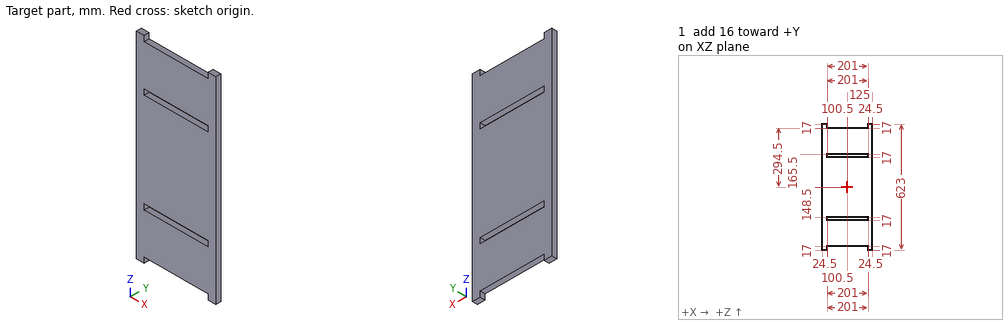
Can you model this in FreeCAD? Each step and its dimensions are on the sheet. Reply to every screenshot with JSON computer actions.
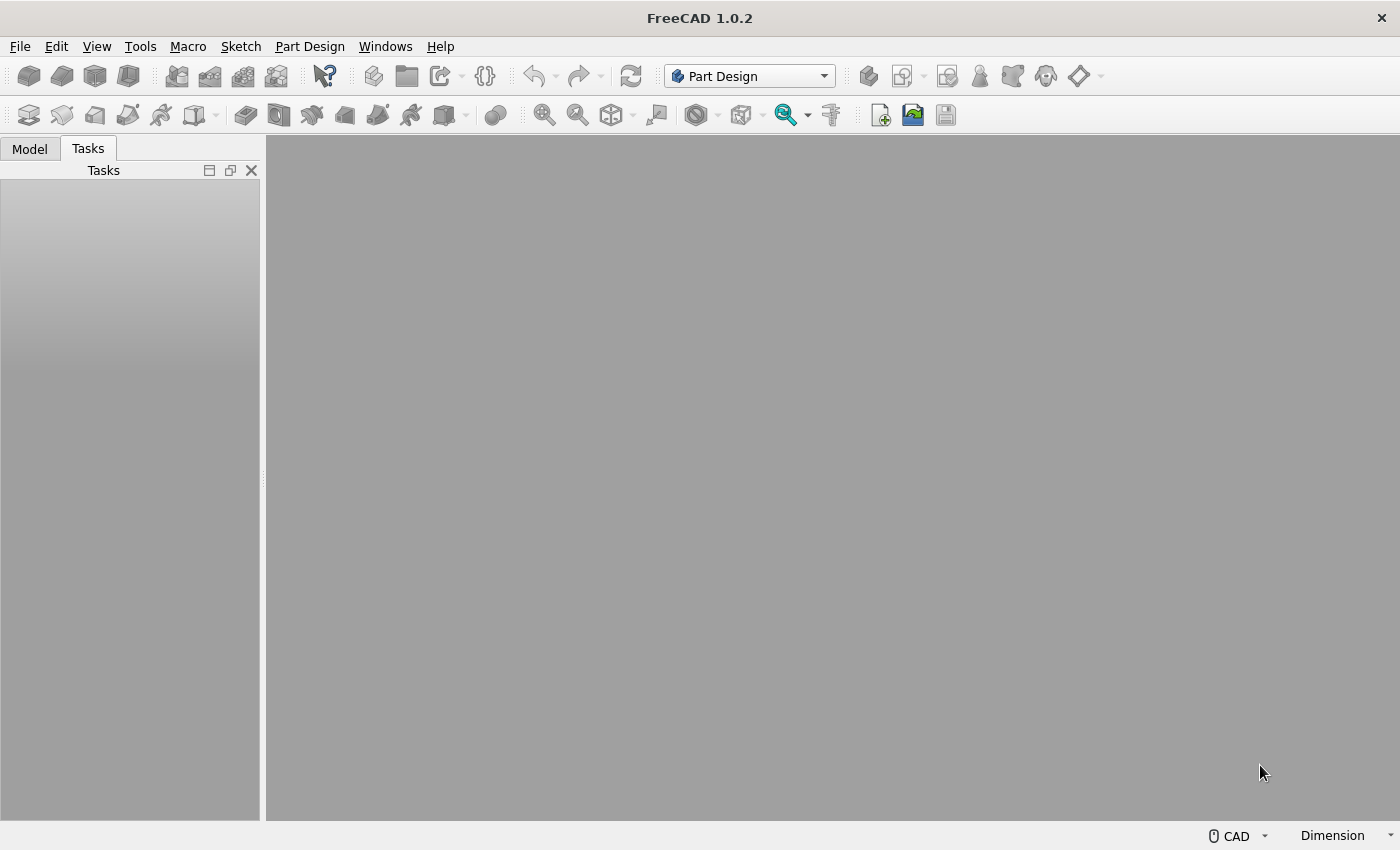
{"action": "left_click", "coordinate": [880, 116]}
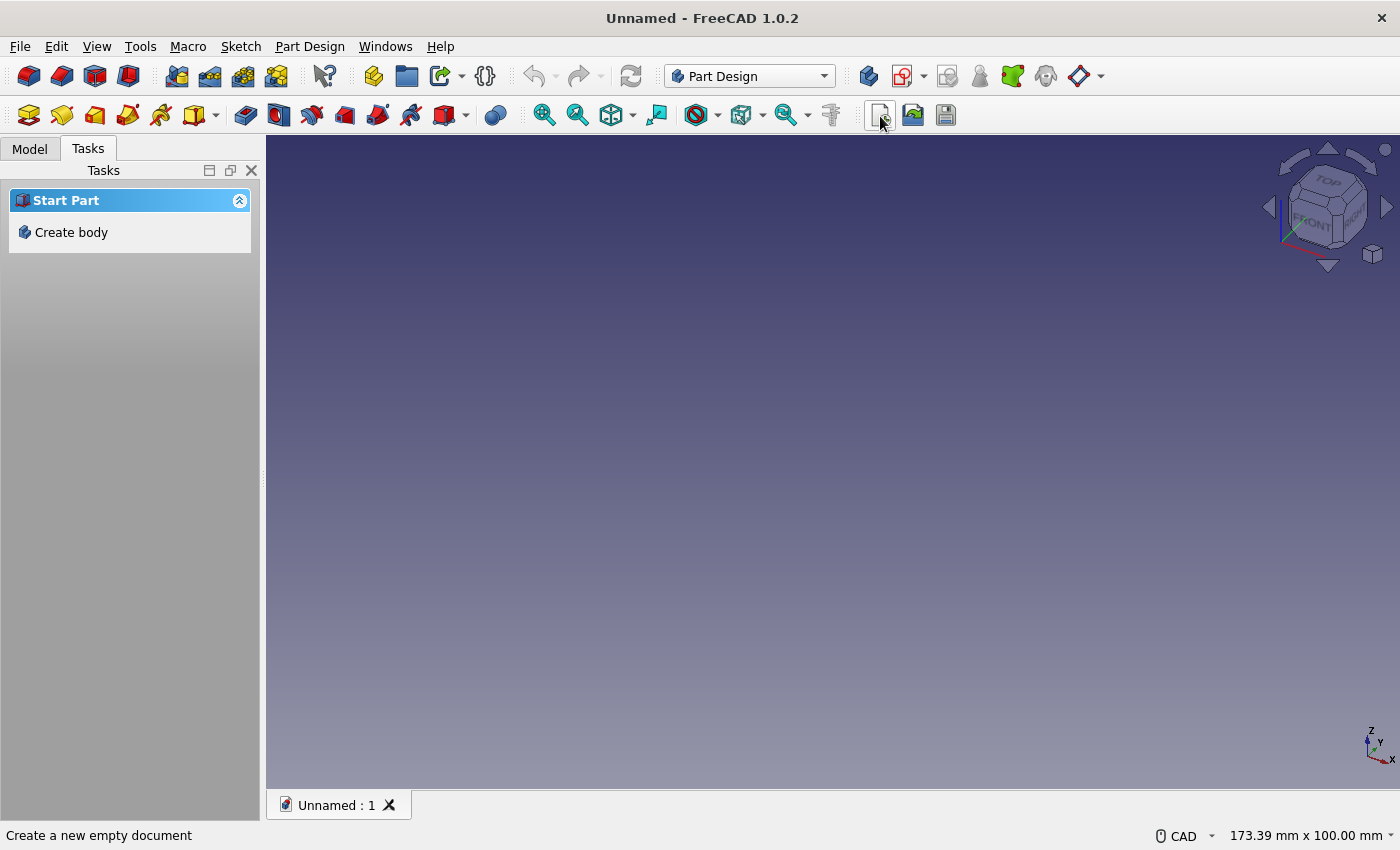
{"action": "left_click", "coordinate": [902, 76]}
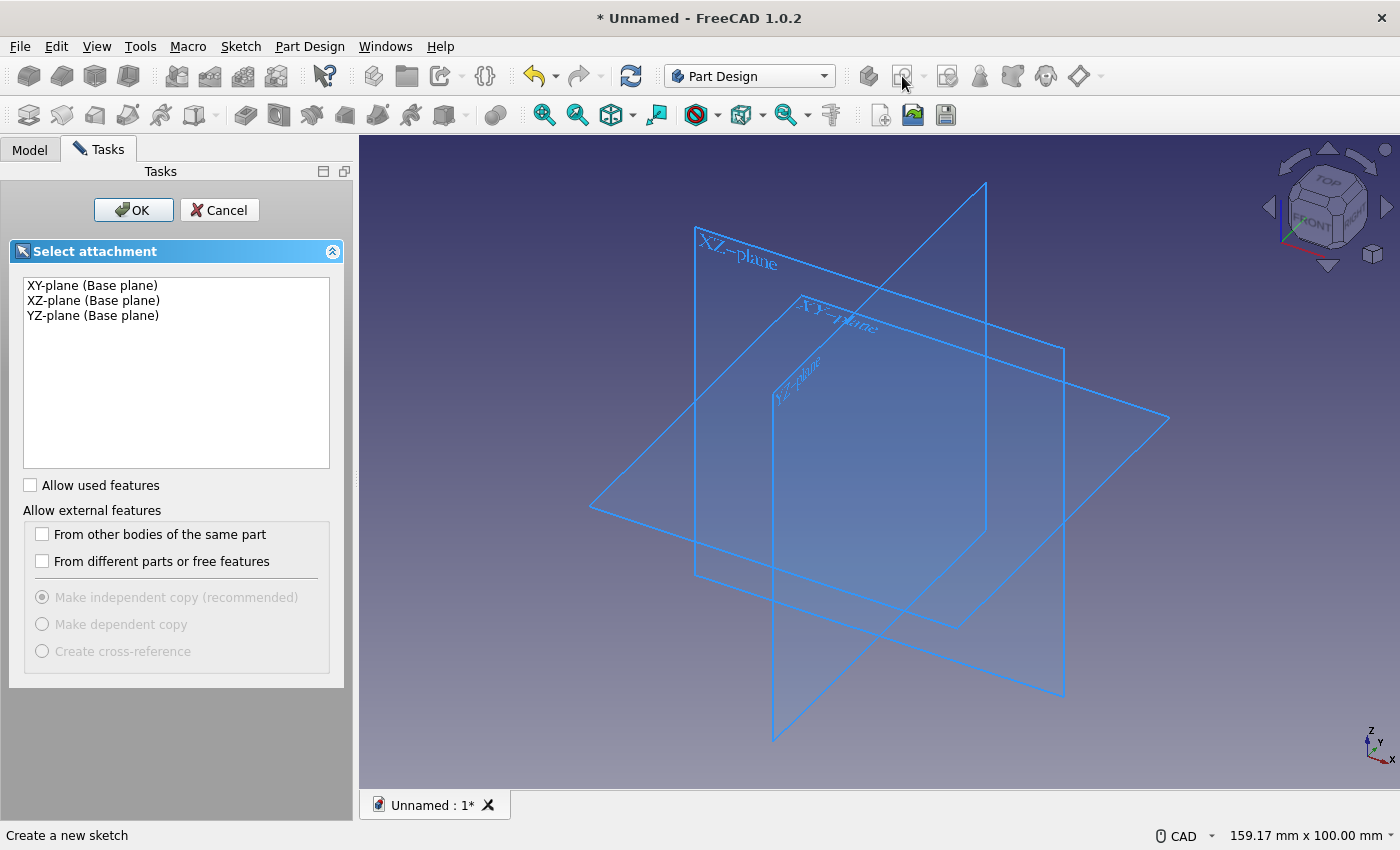
{"action": "left_click", "coordinate": [84, 300]}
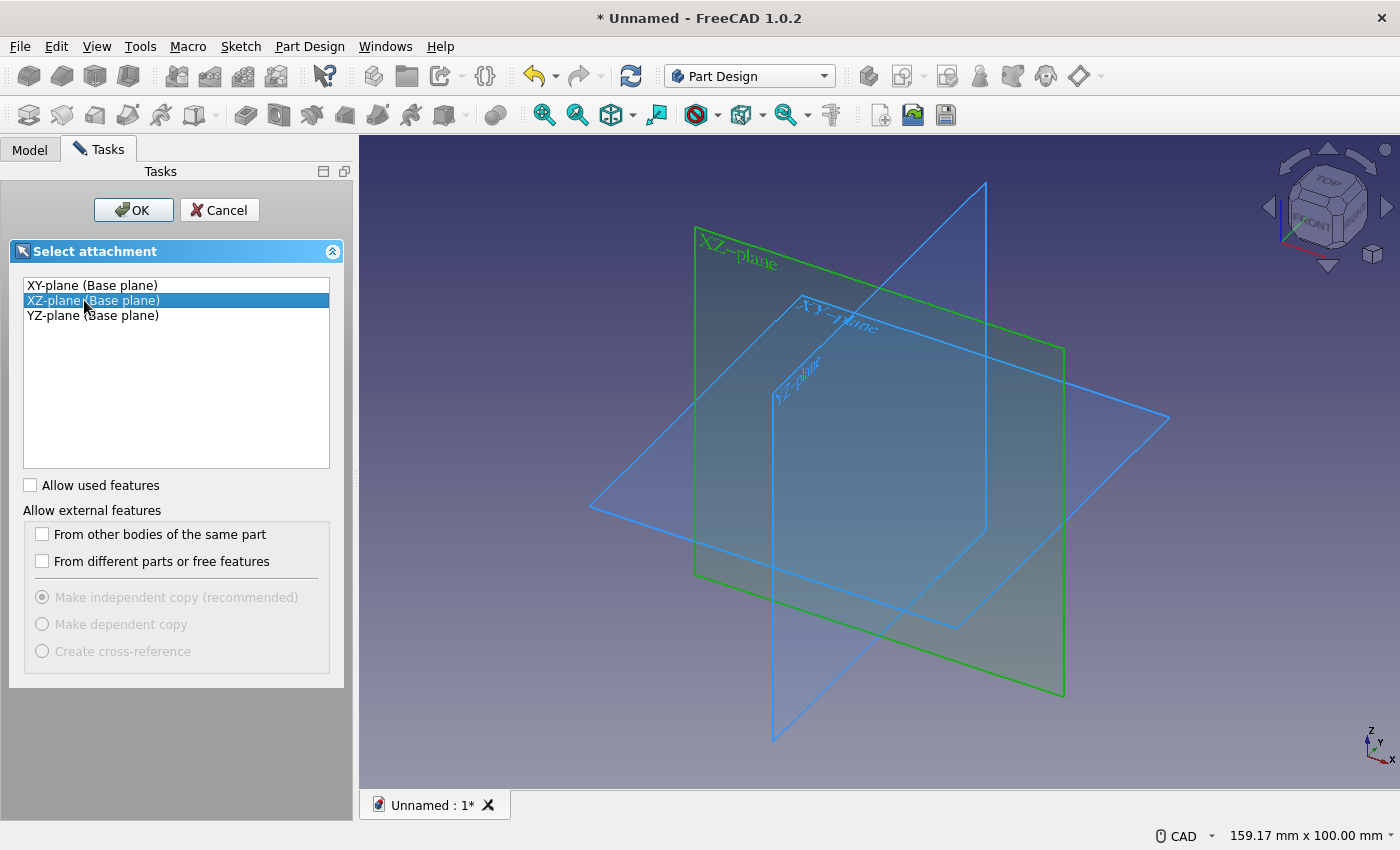
{"action": "left_click", "coordinate": [134, 210]}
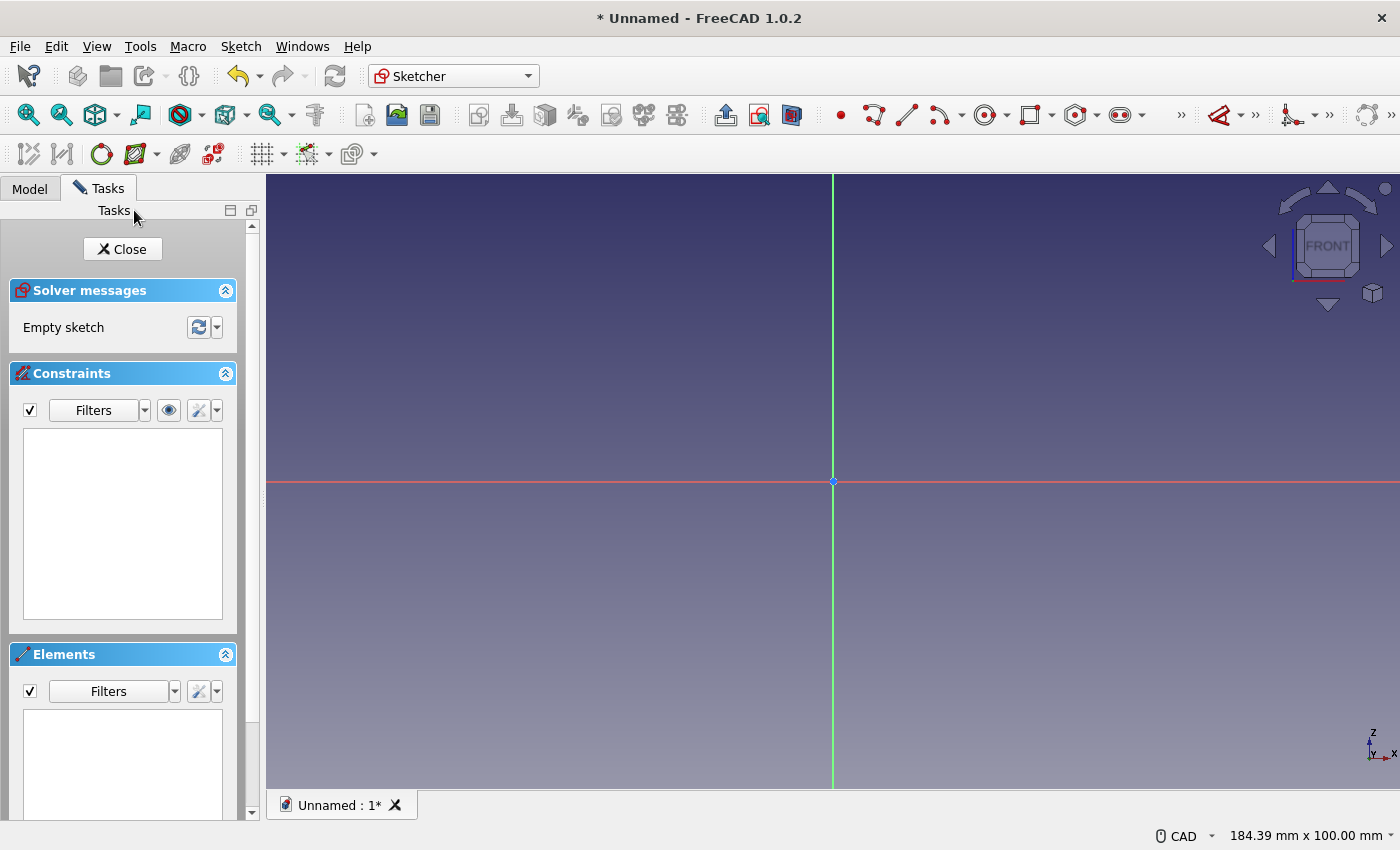
{"action": "scroll", "coordinate": [756, 482], "scroll_direction": "down", "scroll_amount": 11}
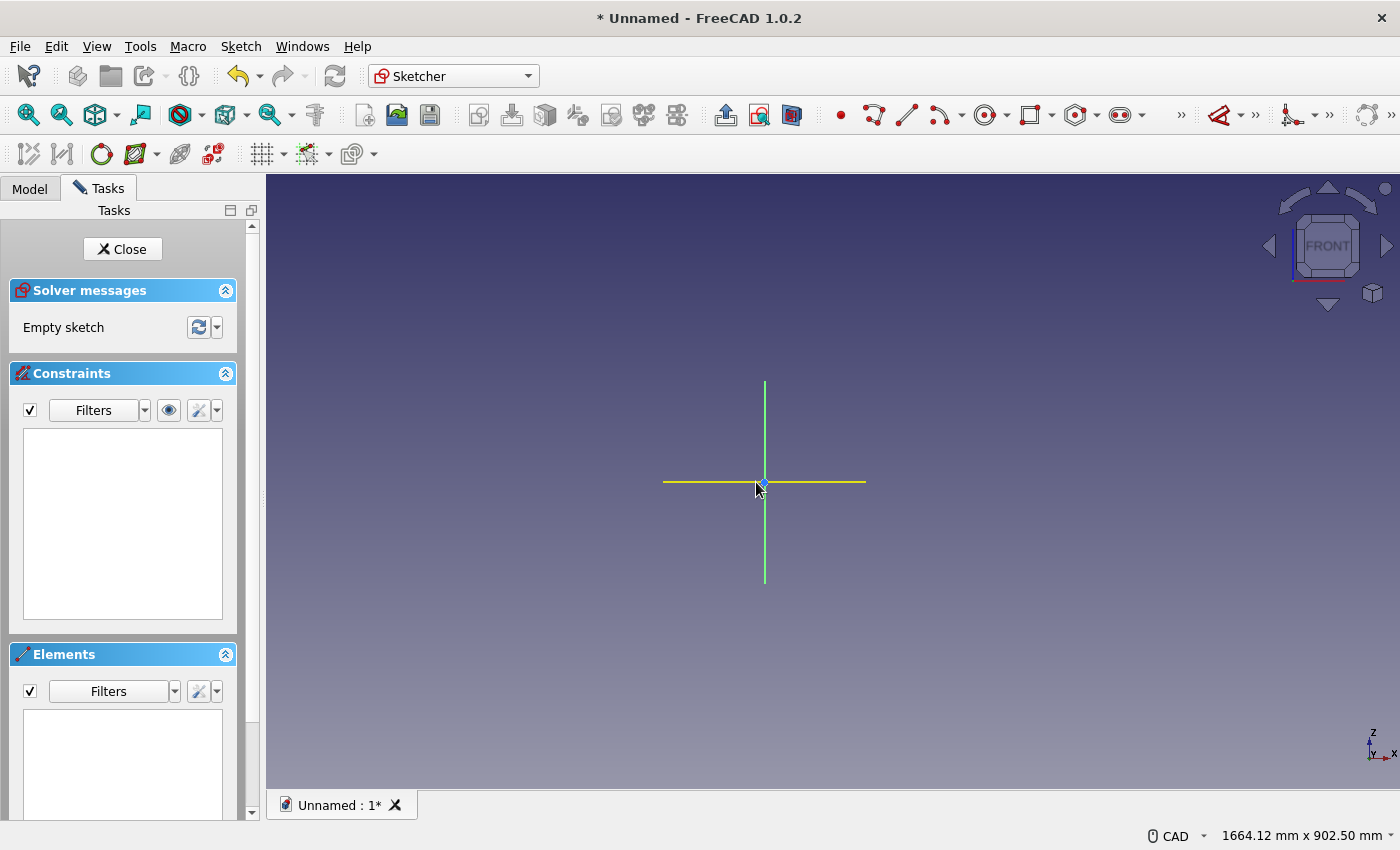
{"action": "left_click", "coordinate": [874, 116]}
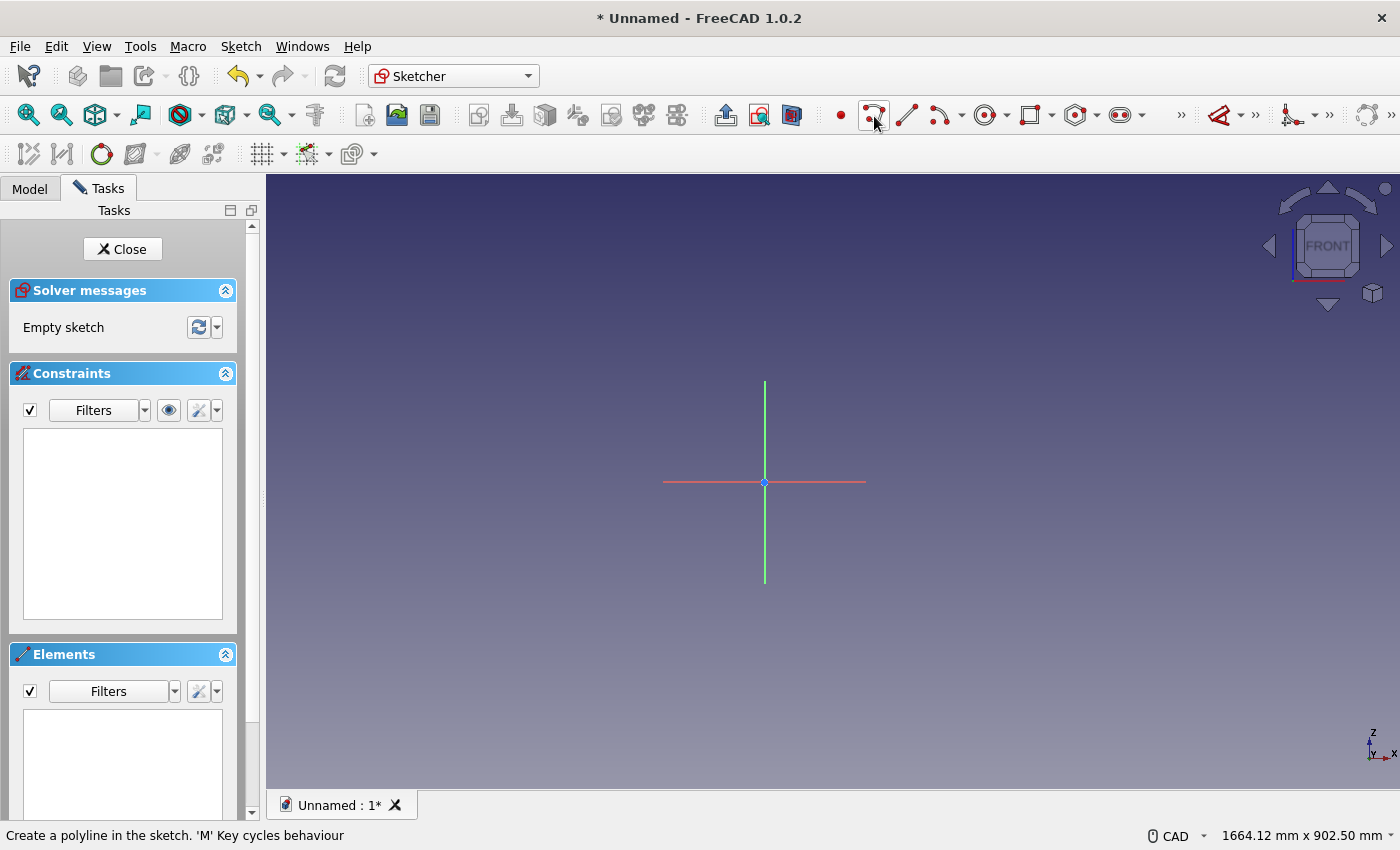
{"action": "left_click", "coordinate": [696, 282]}
{"action": "left_click", "coordinate": [833, 282]}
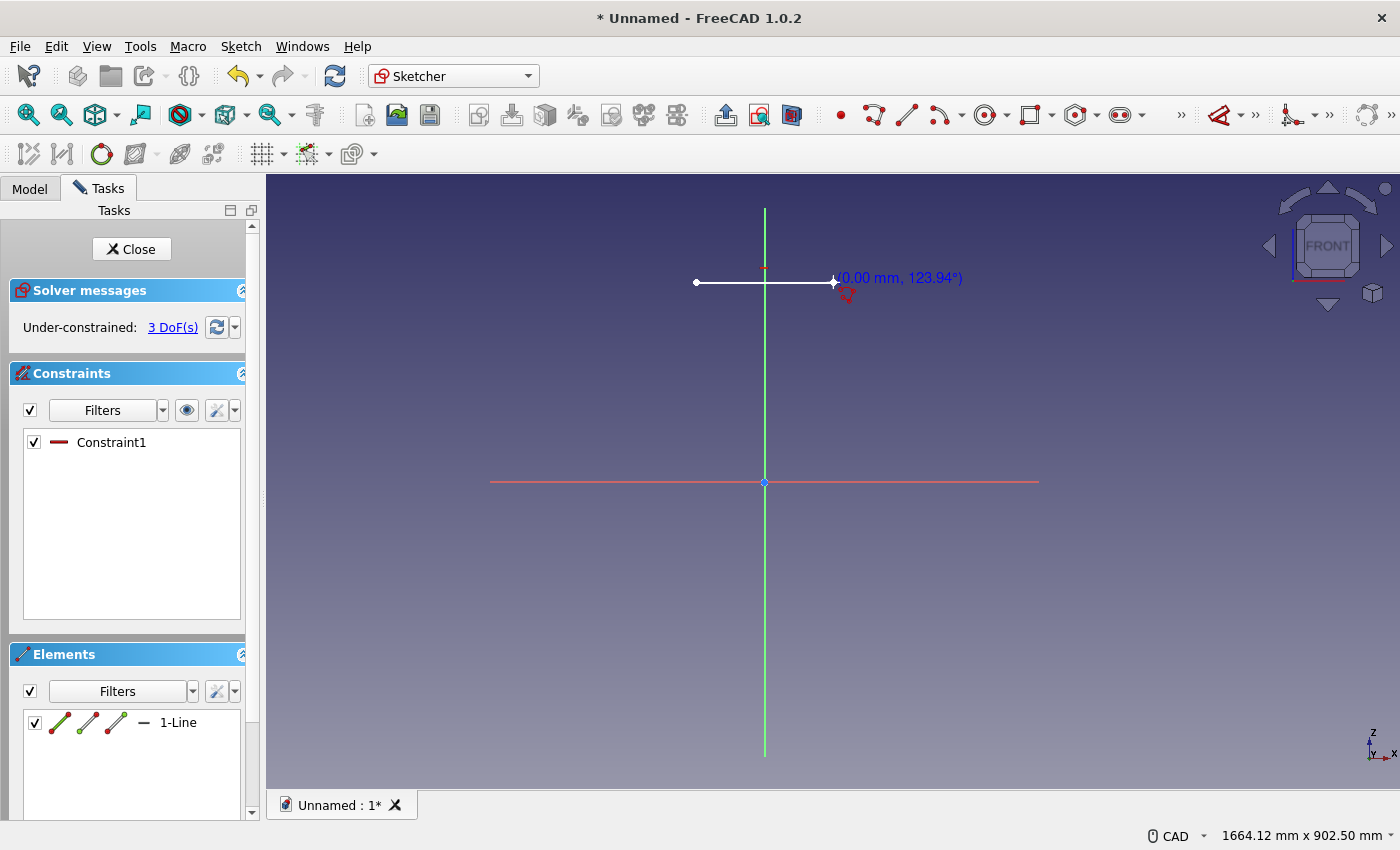
{"action": "scroll", "coordinate": [833, 270], "scroll_direction": "up", "scroll_amount": 2}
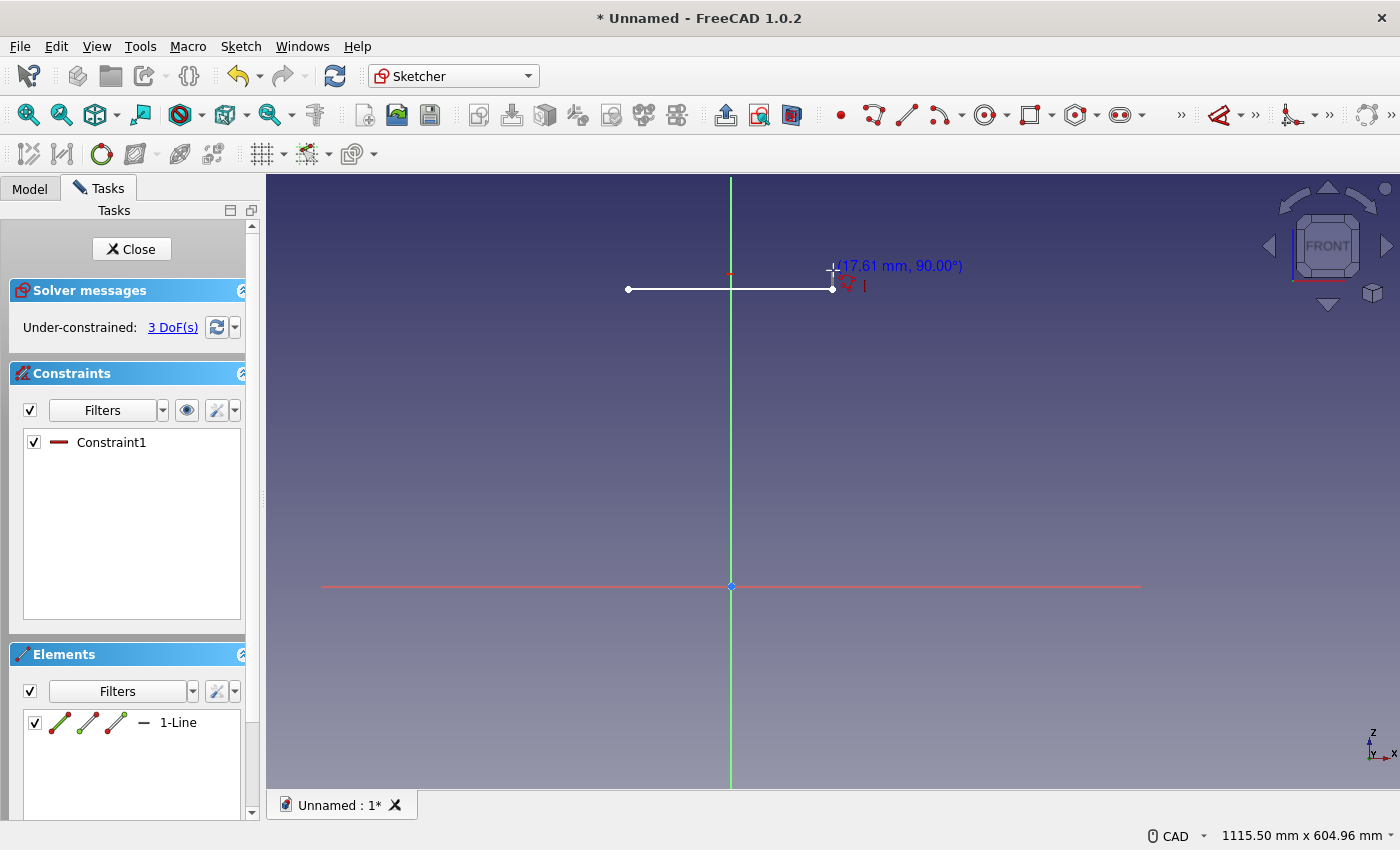
{"action": "left_click", "coordinate": [833, 270]}
{"action": "left_click", "coordinate": [858, 270]}